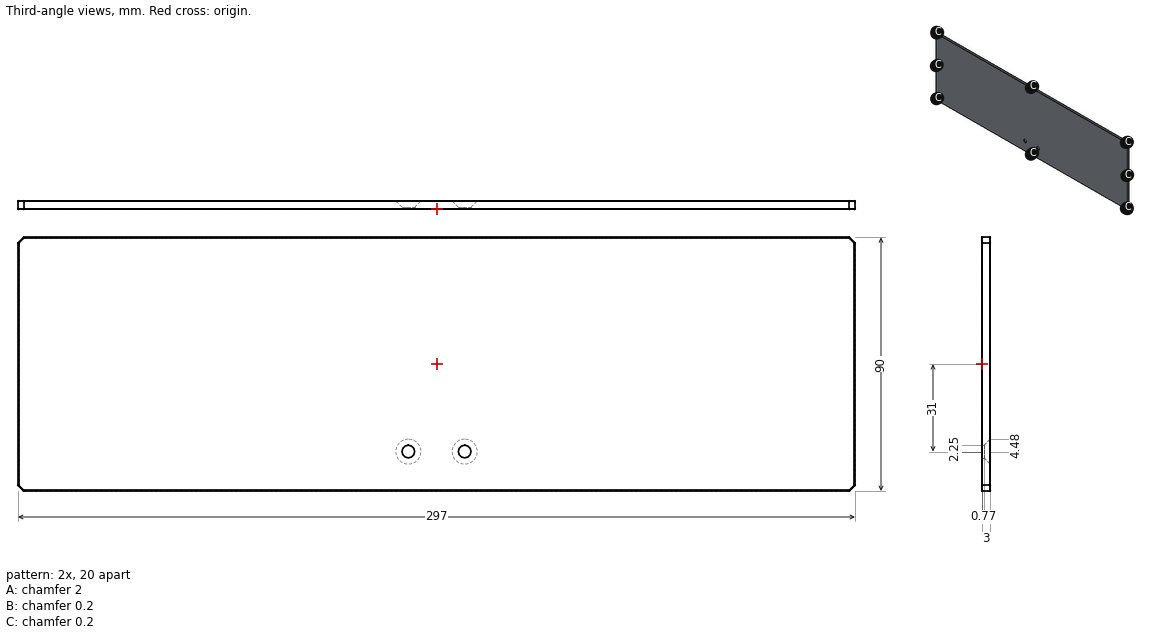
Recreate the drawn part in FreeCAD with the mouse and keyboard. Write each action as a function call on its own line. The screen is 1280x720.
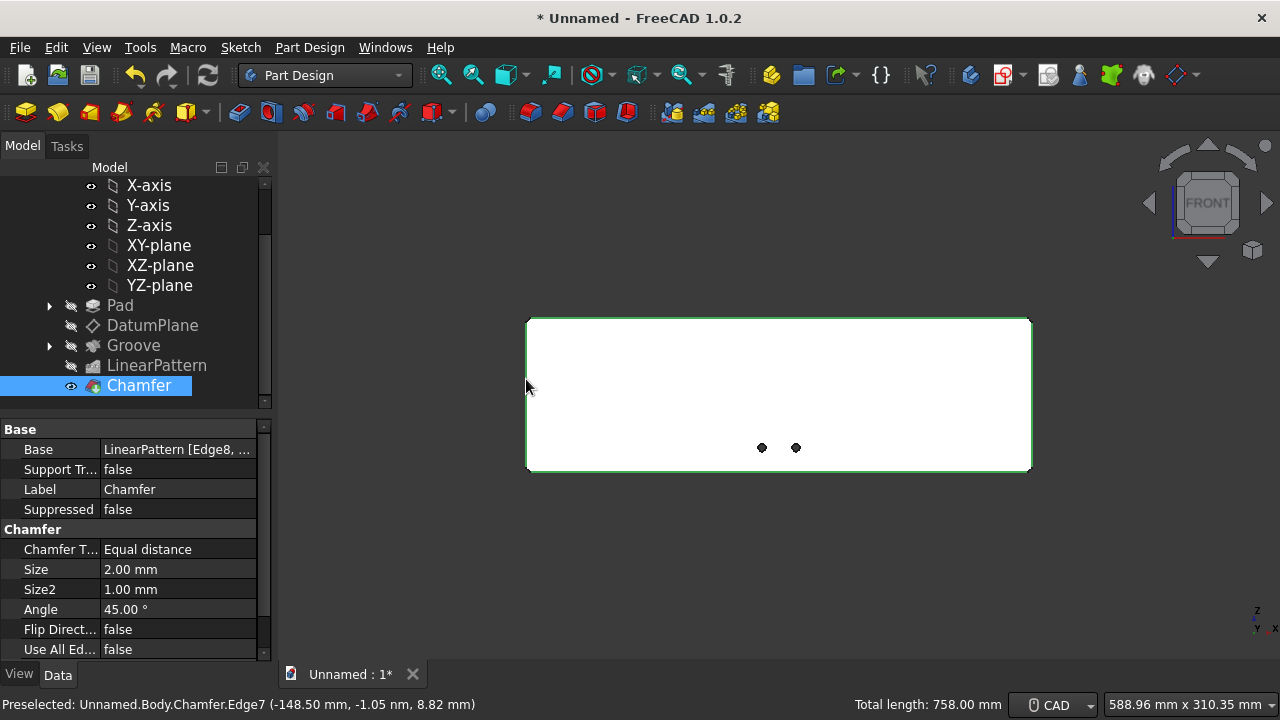
scroll(528, 469, up, 11)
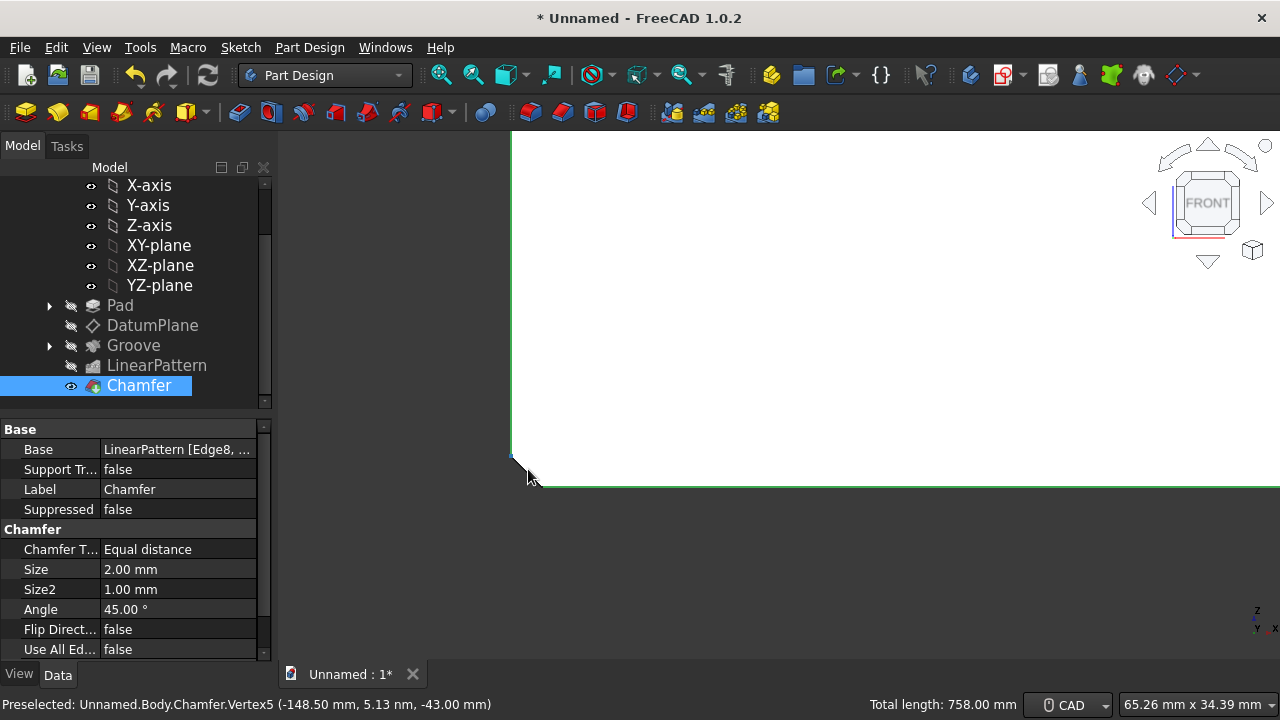
key(v)
key(f)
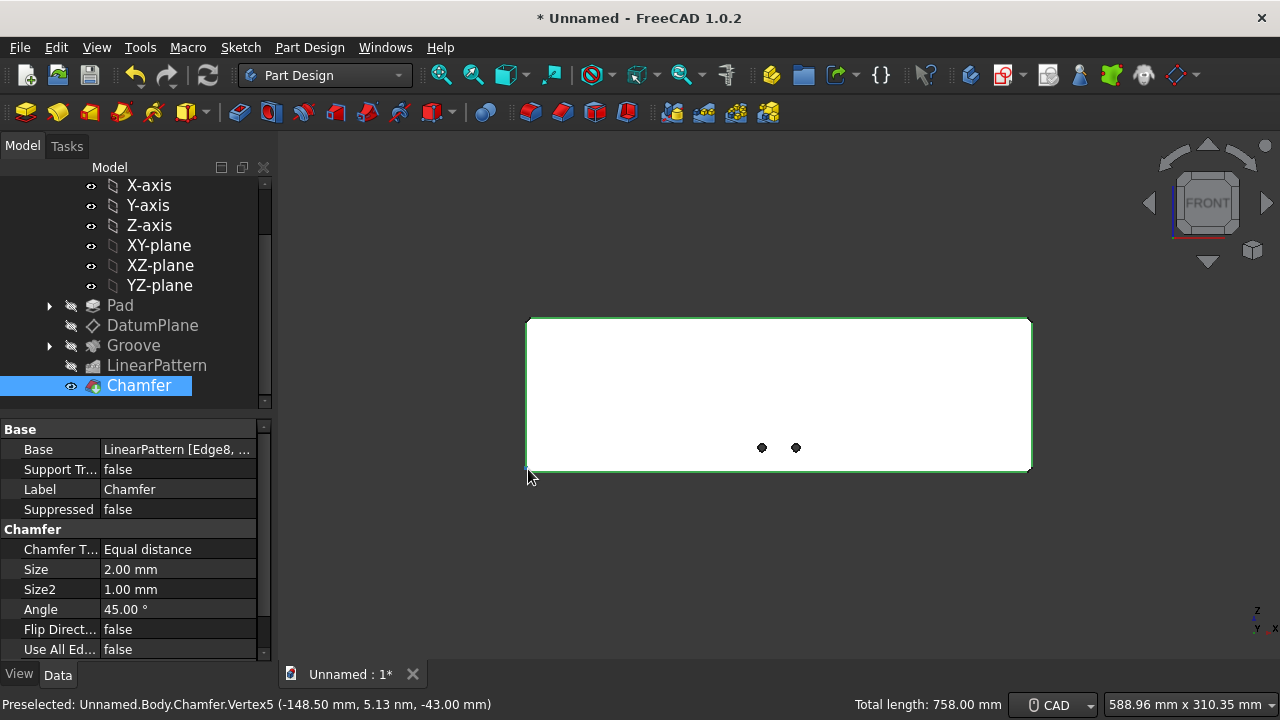
key(3)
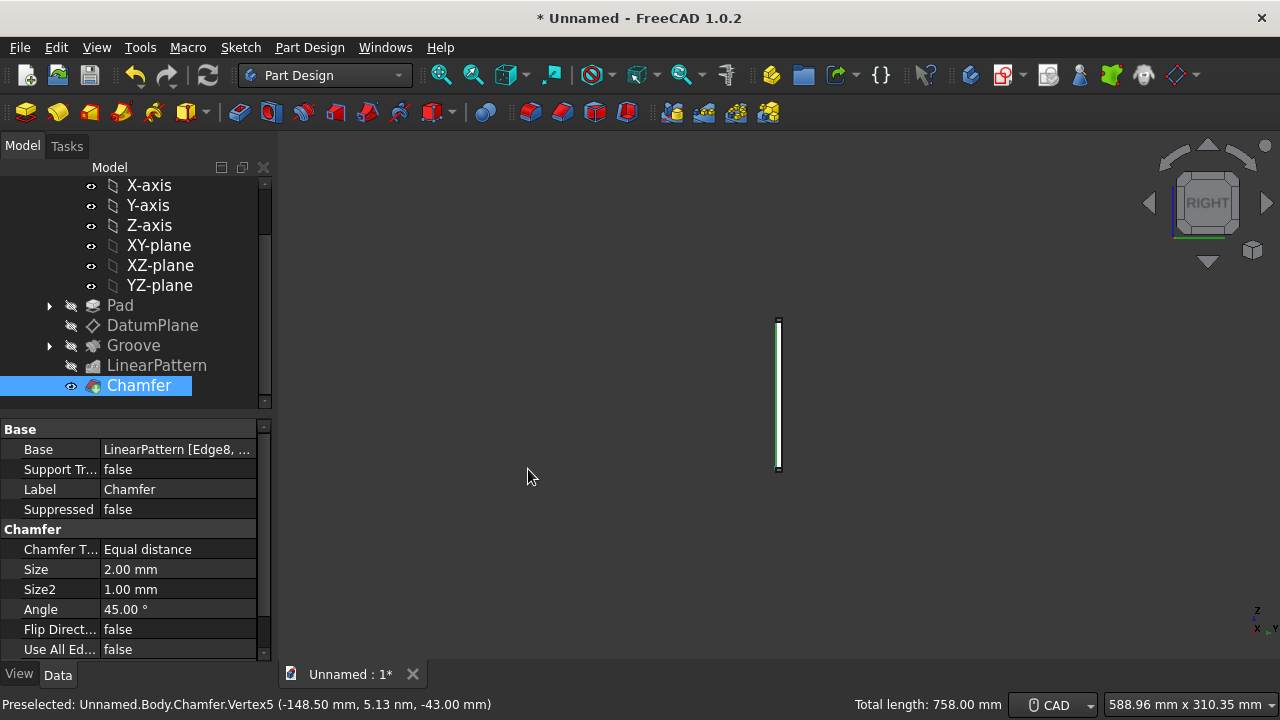
click(442, 76)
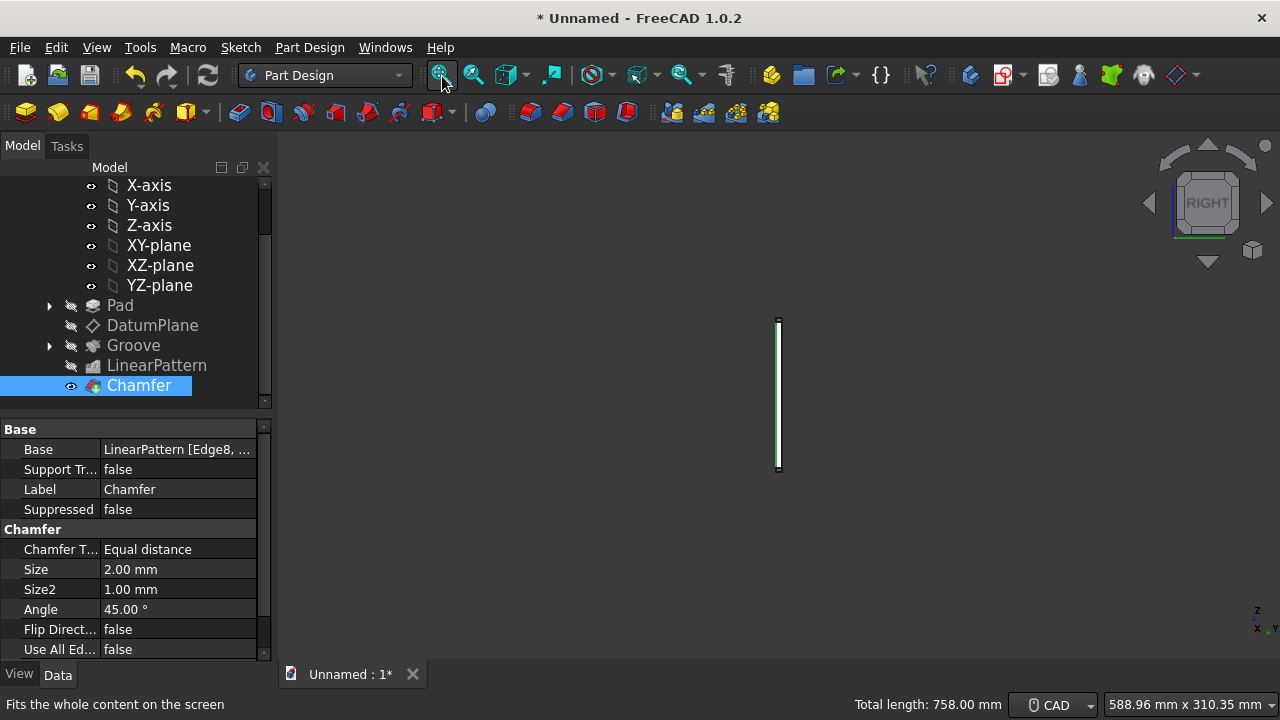
scroll(776, 469, up, 11)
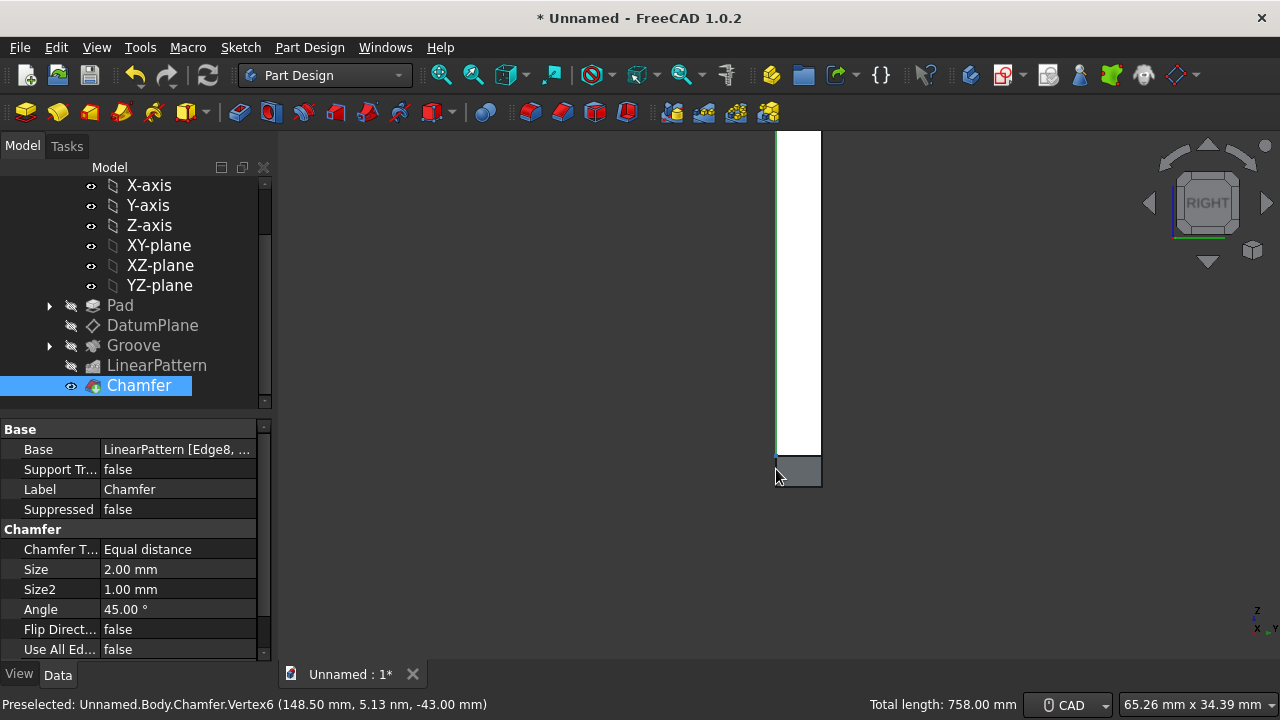
click(776, 471, ctrl)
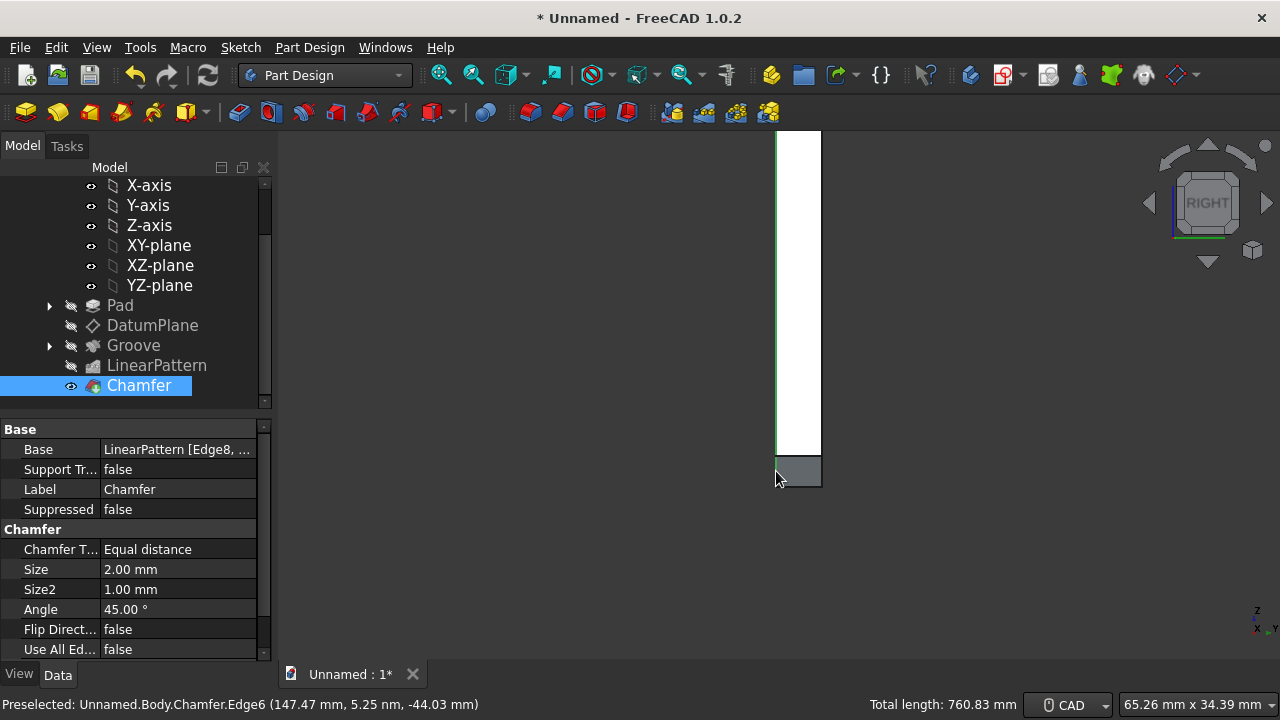
key(v)
key(f)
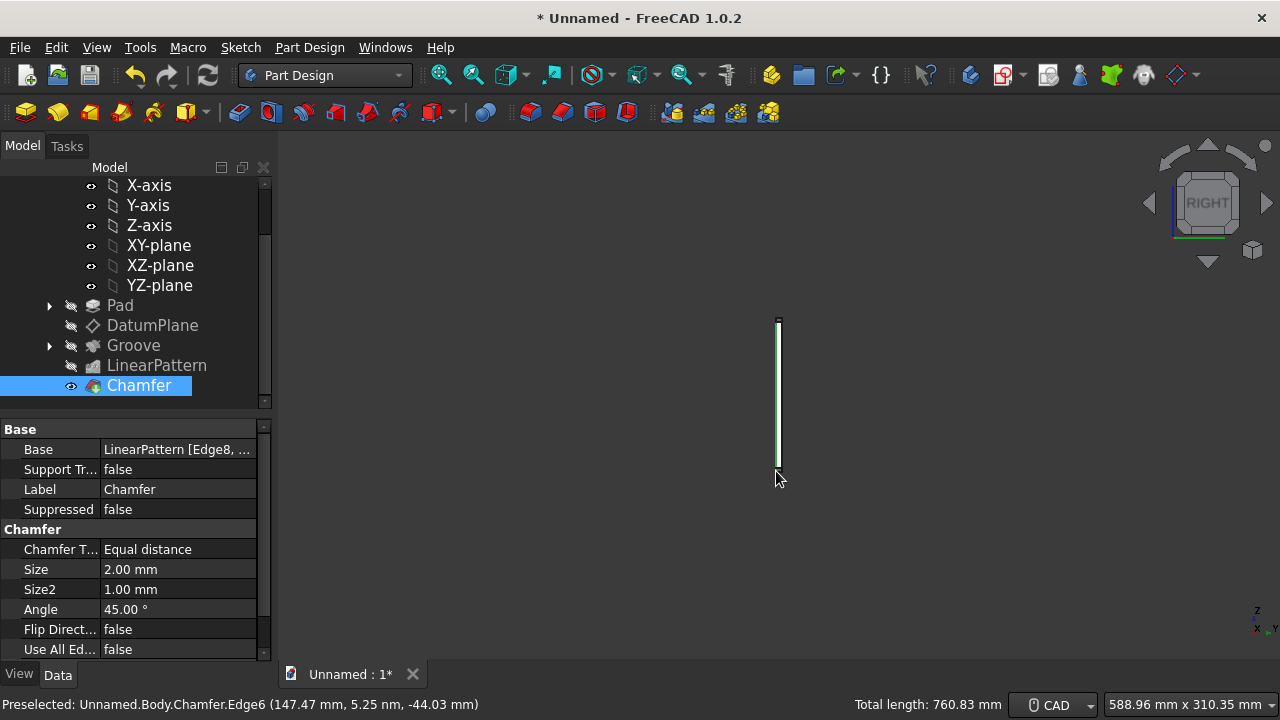
key(5)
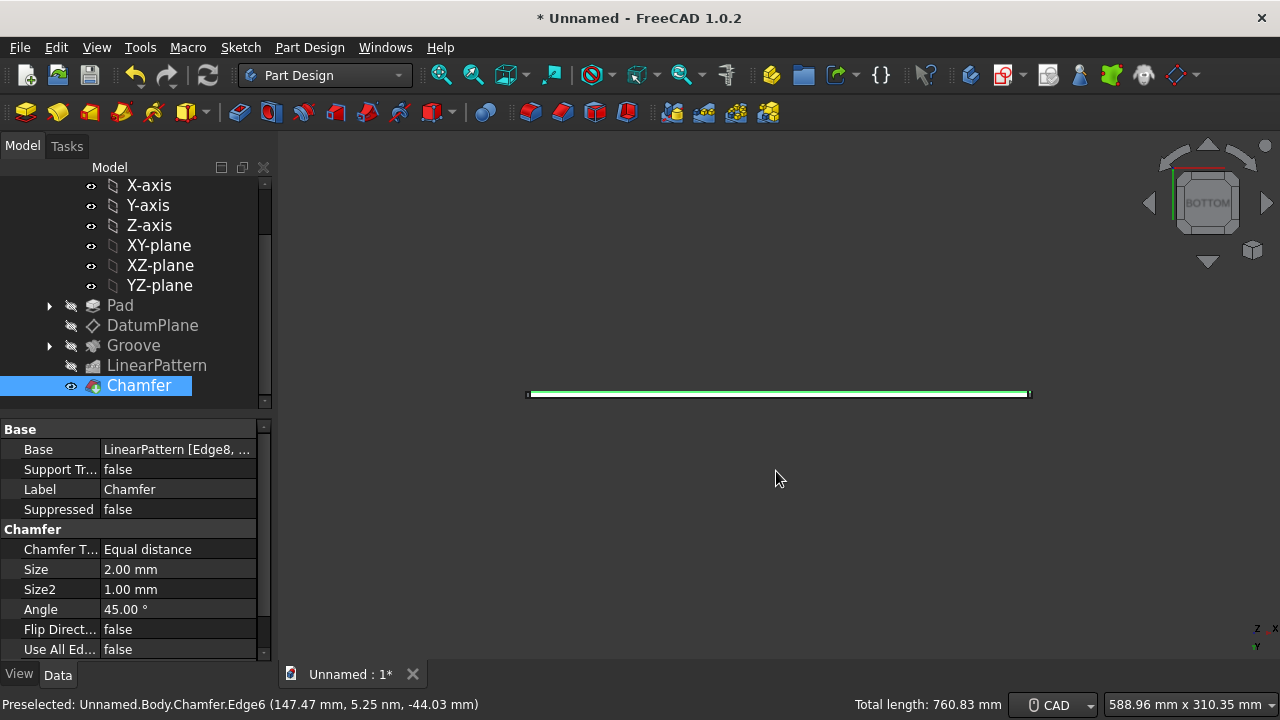
scroll(528, 391, up, 11)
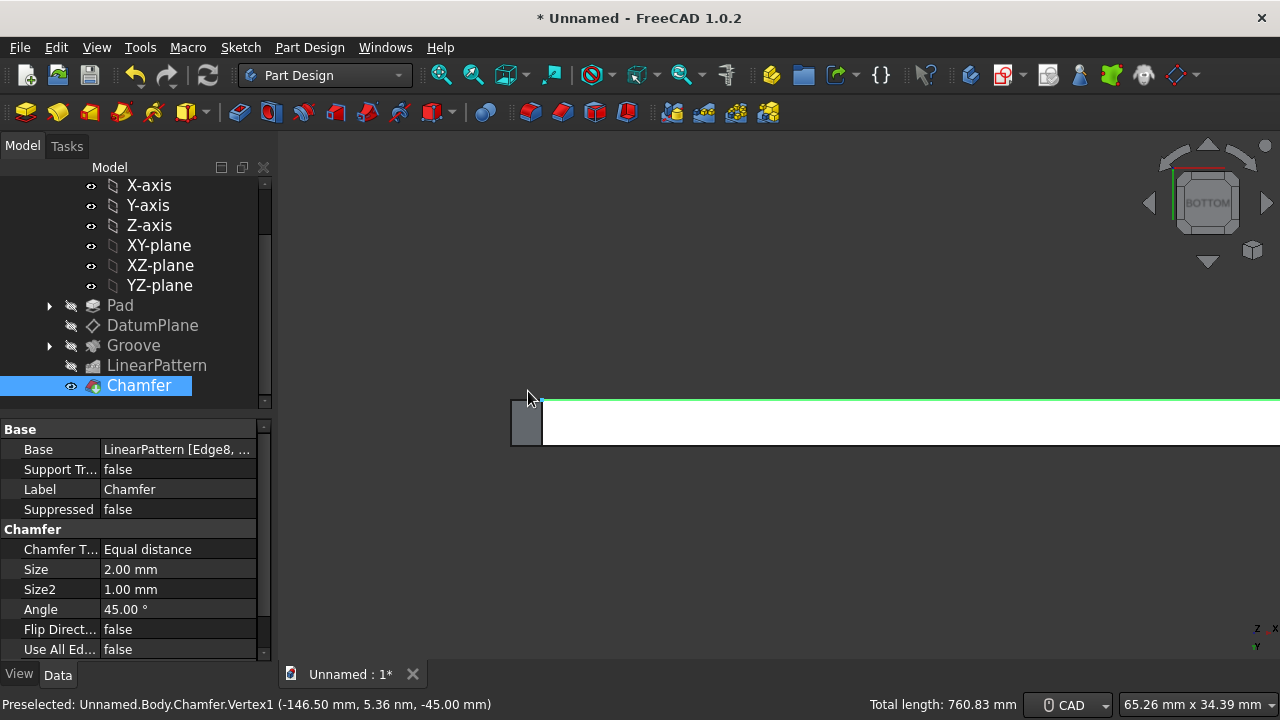
click(527, 399, ctrl)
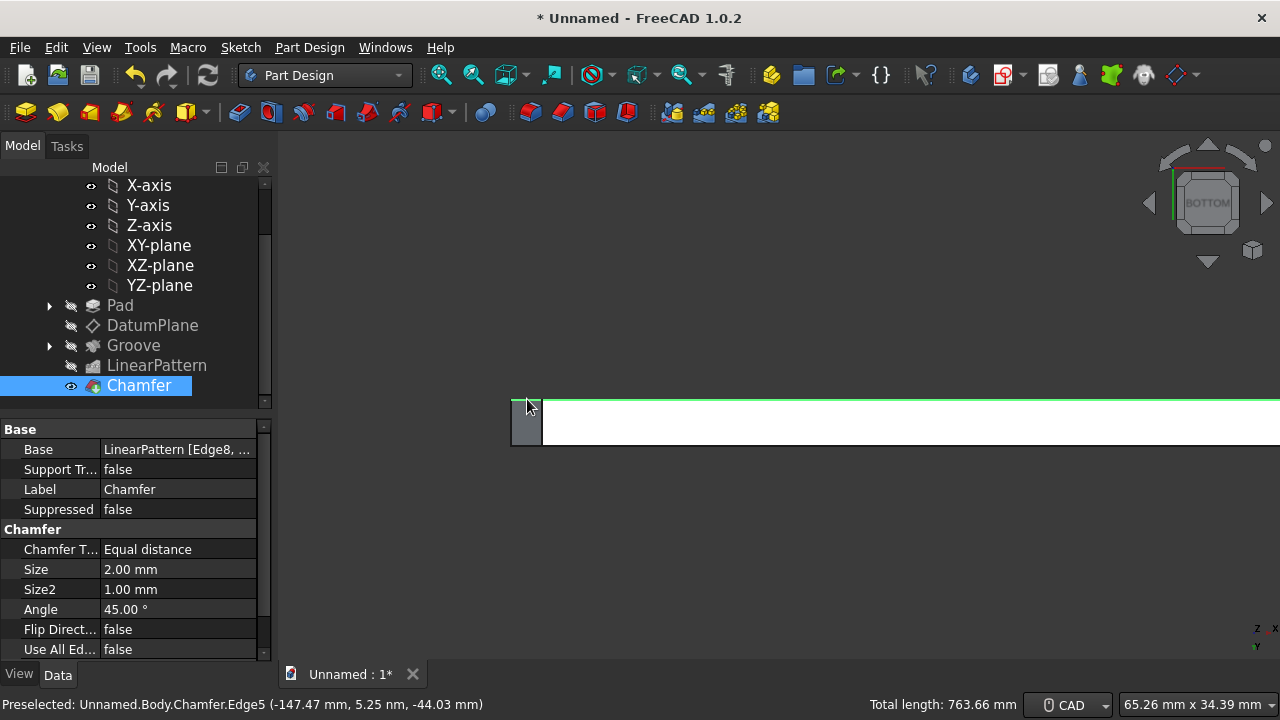
click(442, 76)